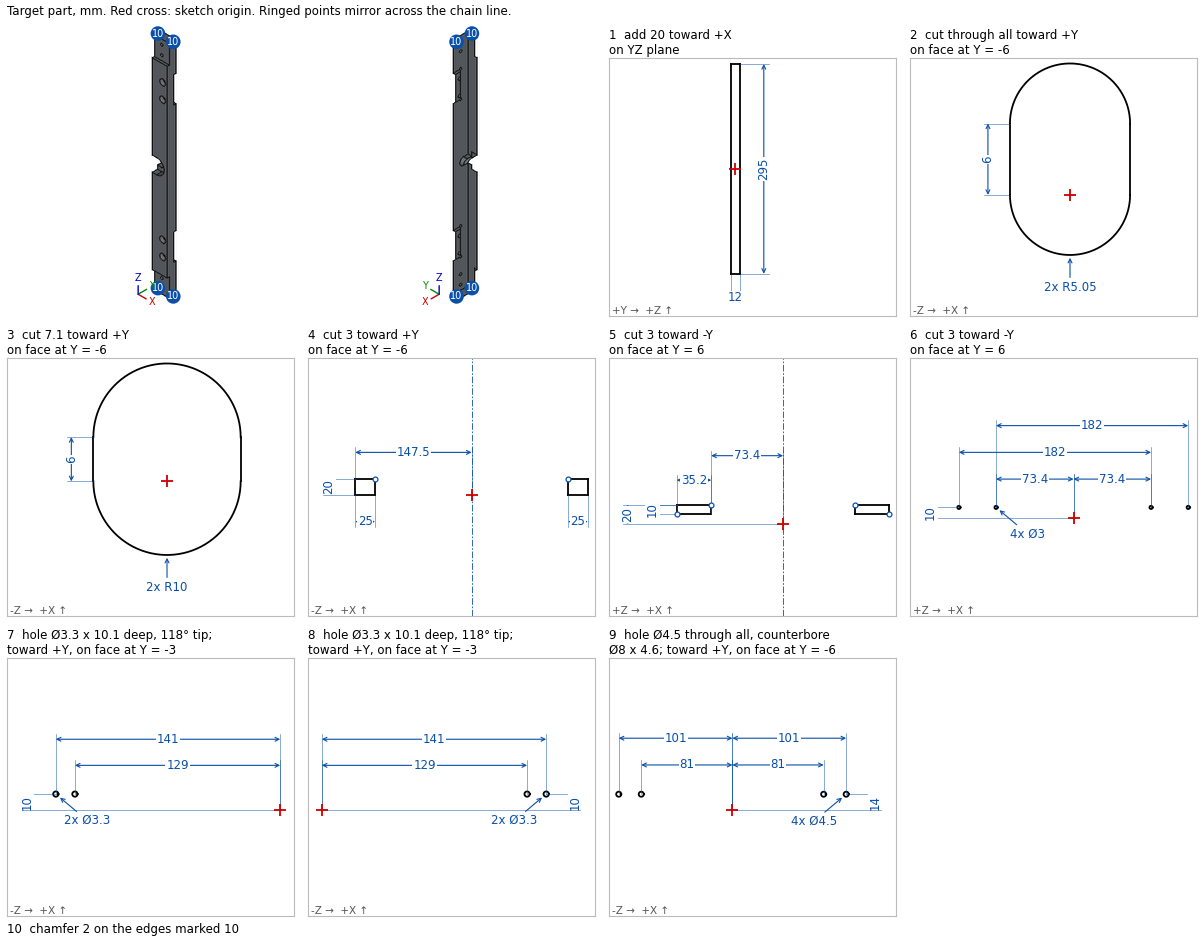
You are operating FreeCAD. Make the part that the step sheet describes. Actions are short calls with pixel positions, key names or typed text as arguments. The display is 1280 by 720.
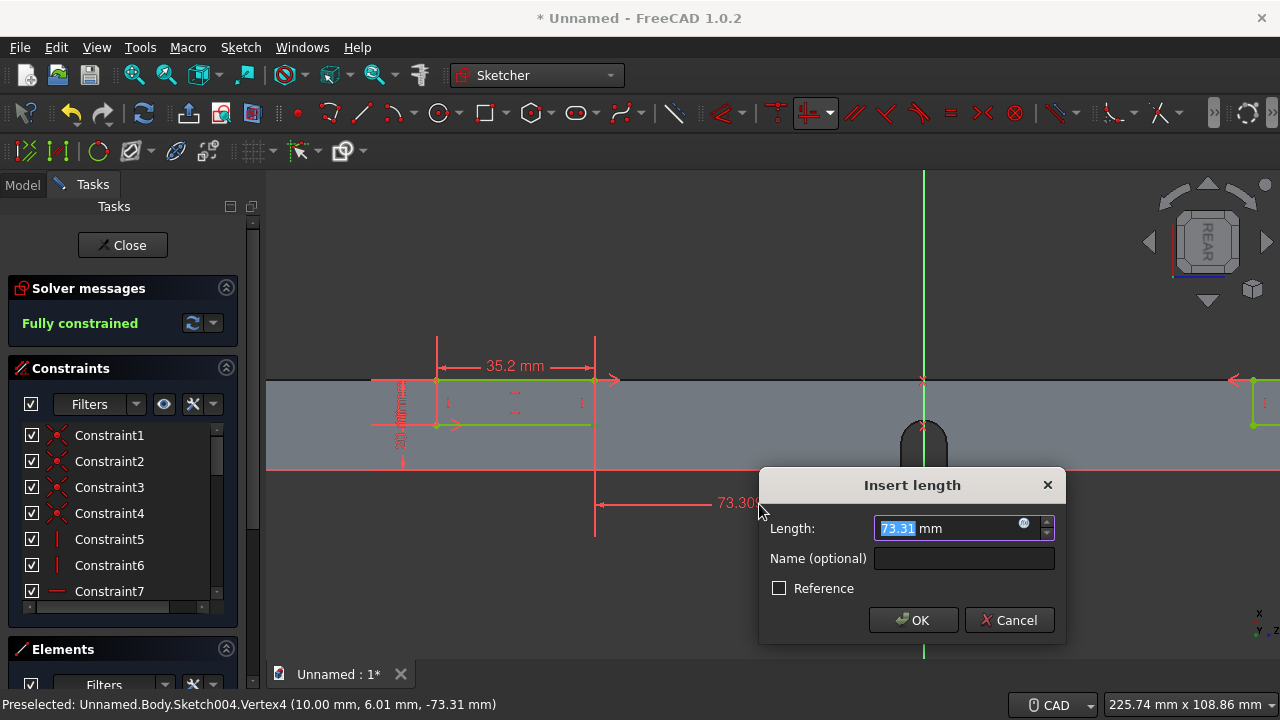
text(73.4)
key(Return)
key(Escape)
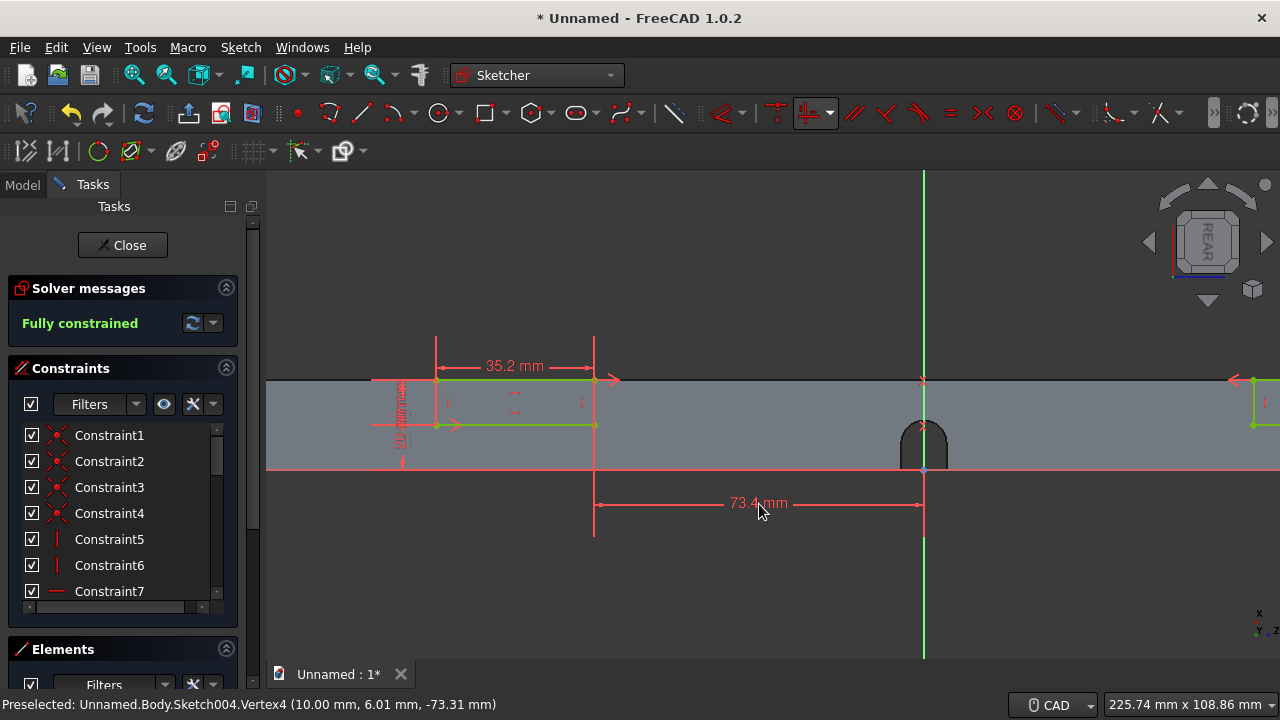
click(123, 245)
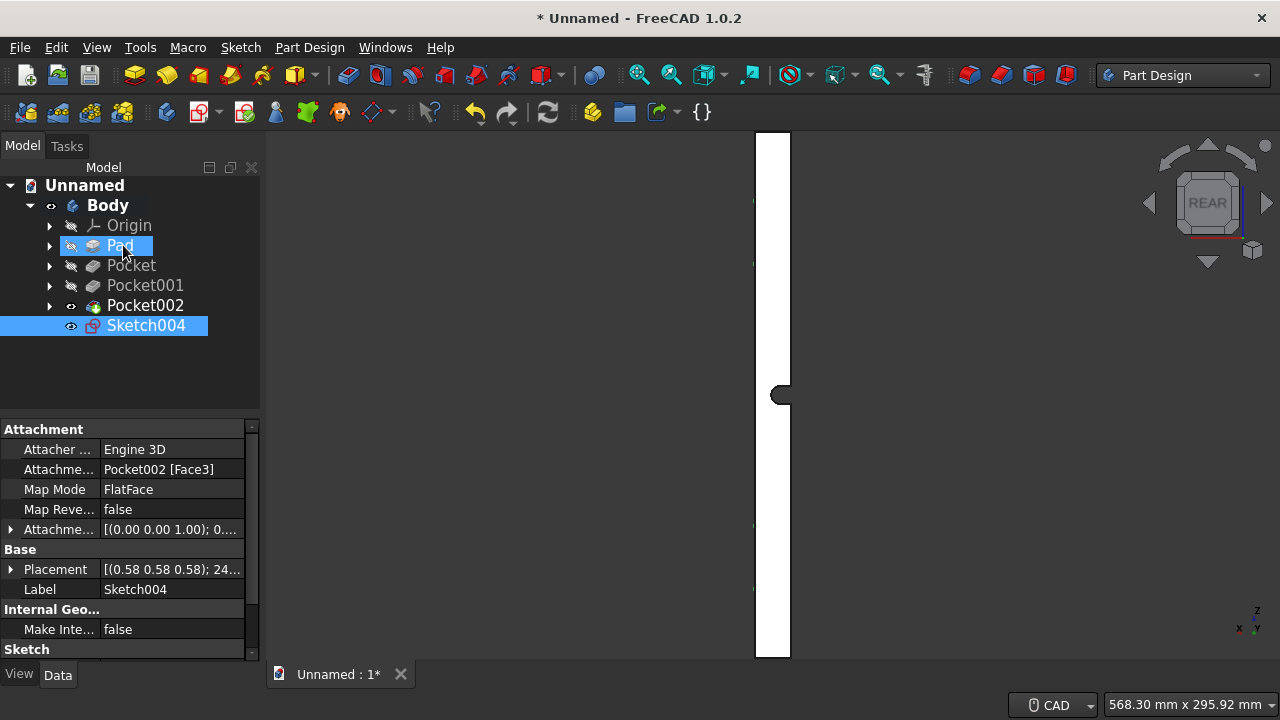
click(350, 76)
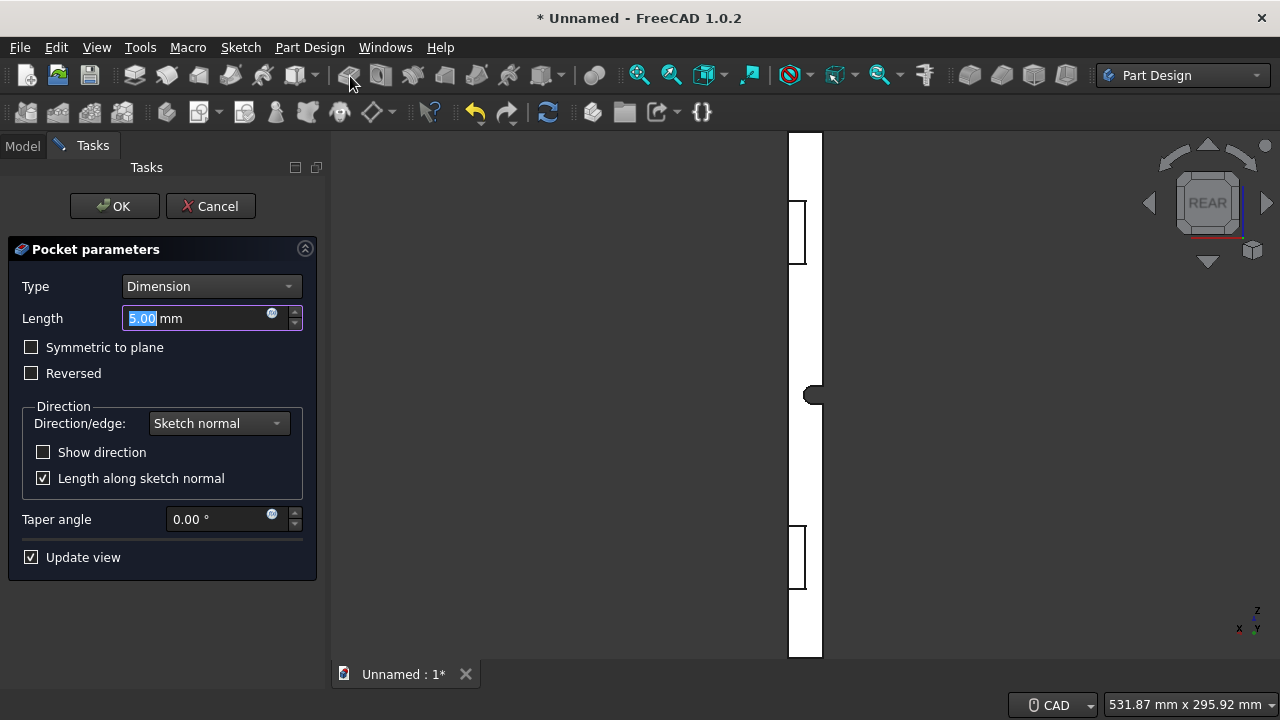
text(3)
key(Tab)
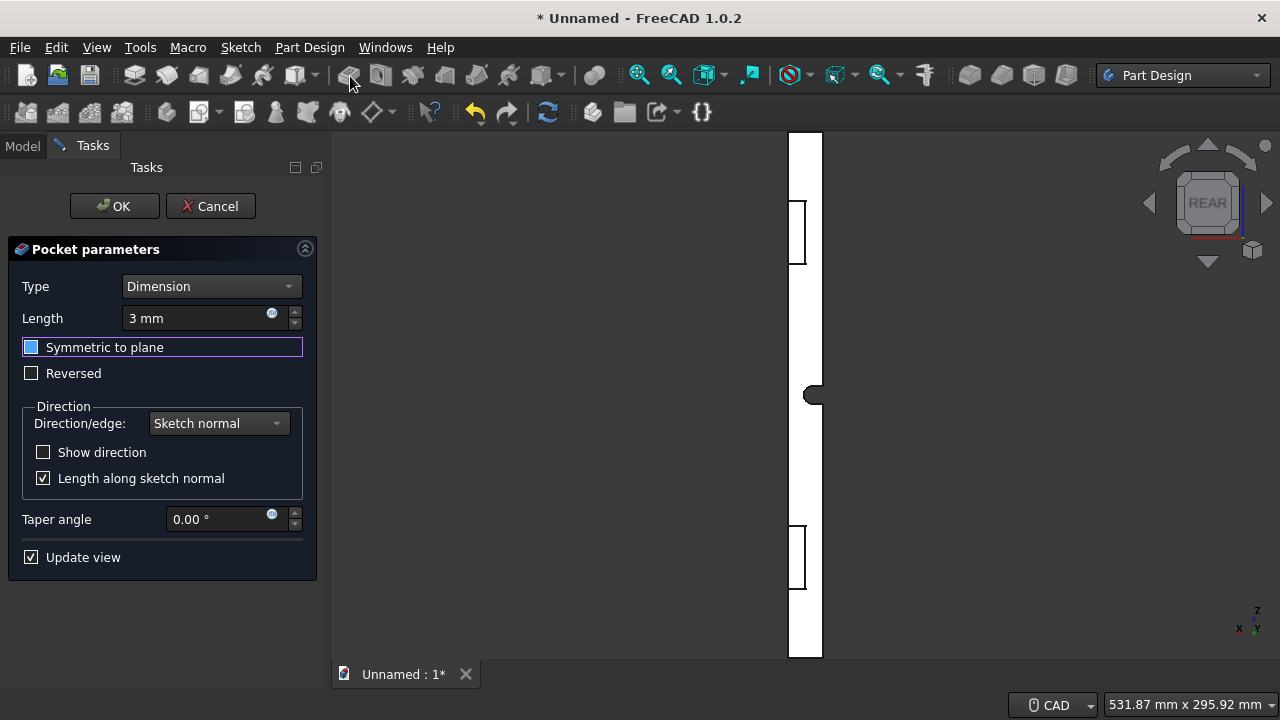
click(115, 206)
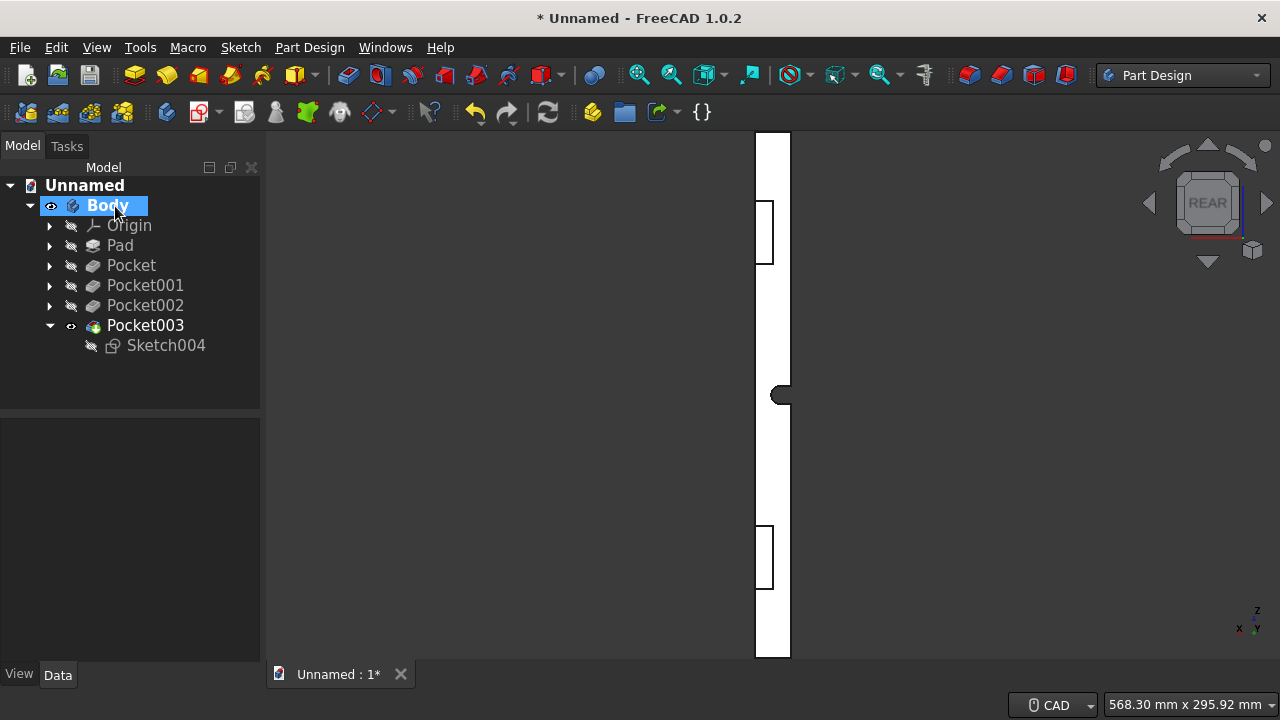
click(773, 469)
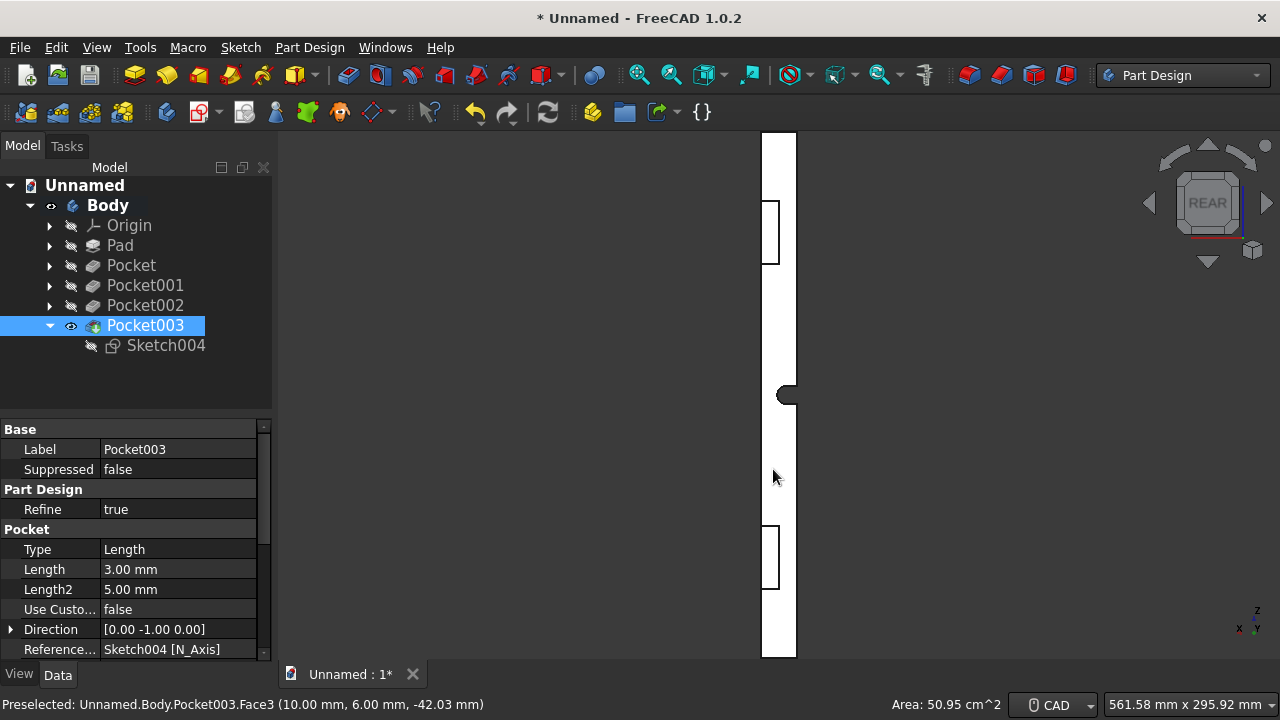
click(200, 112)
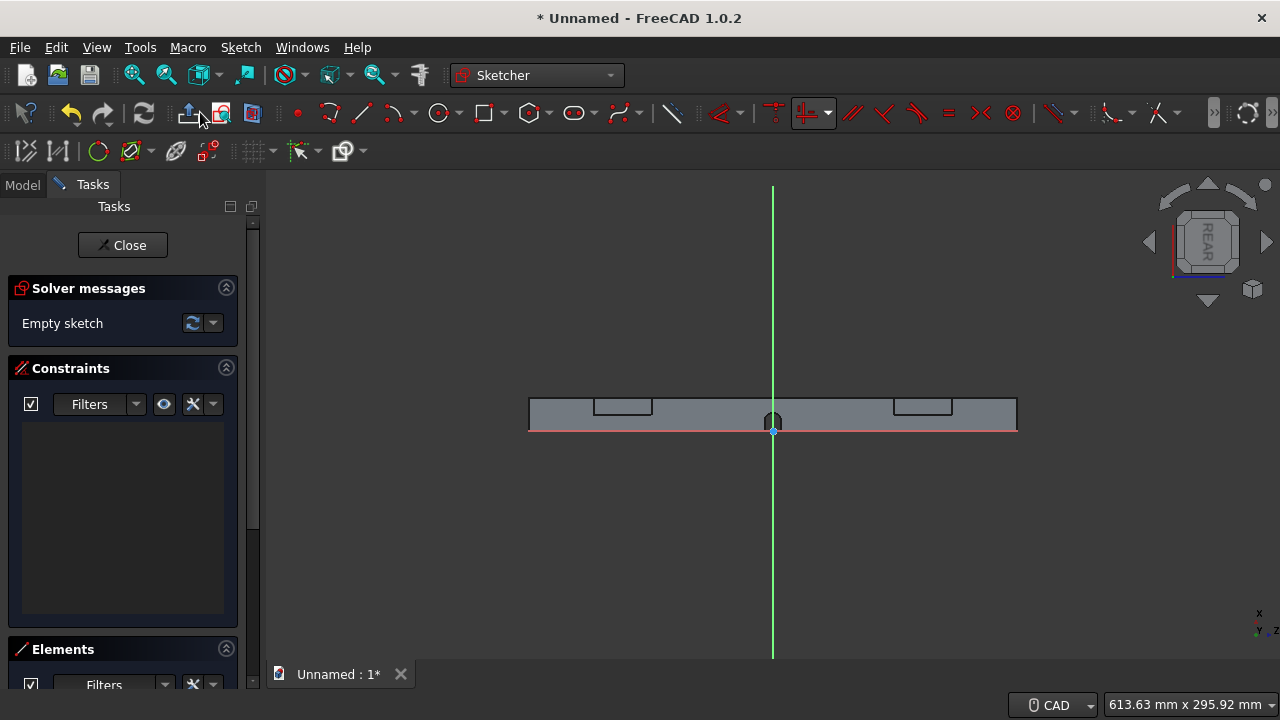
scroll(912, 436, up, 2)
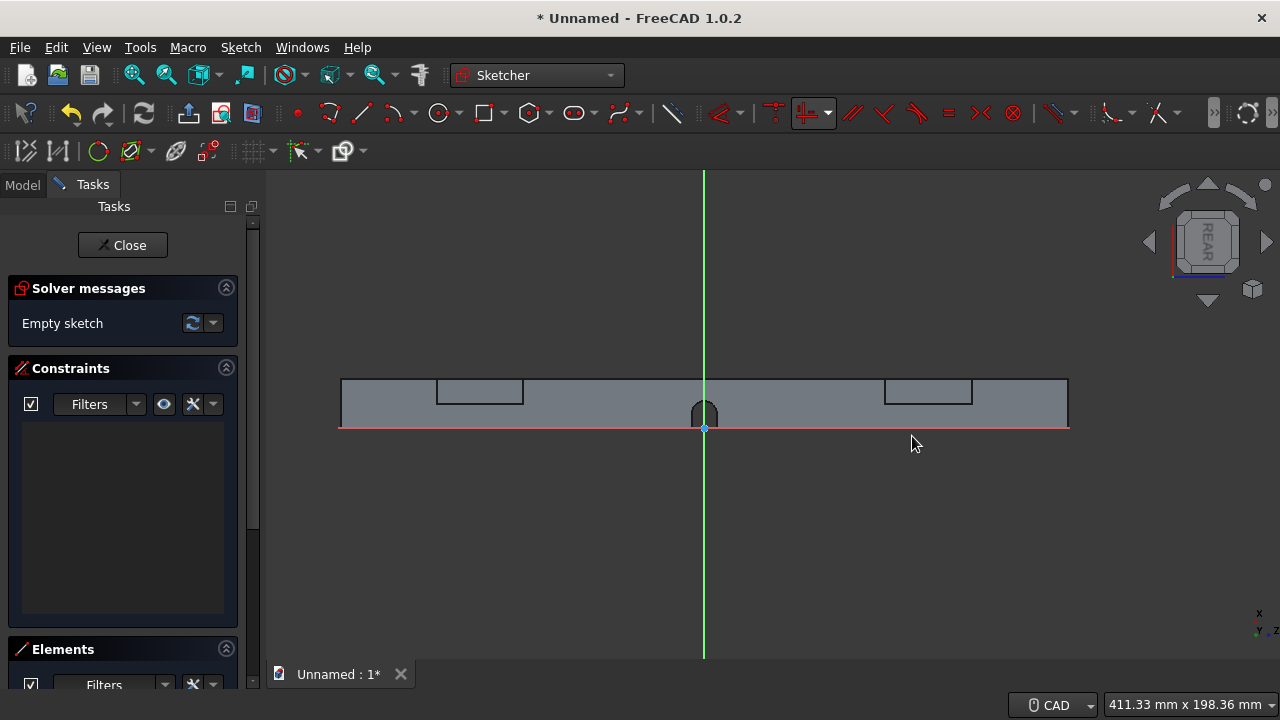
click(440, 114)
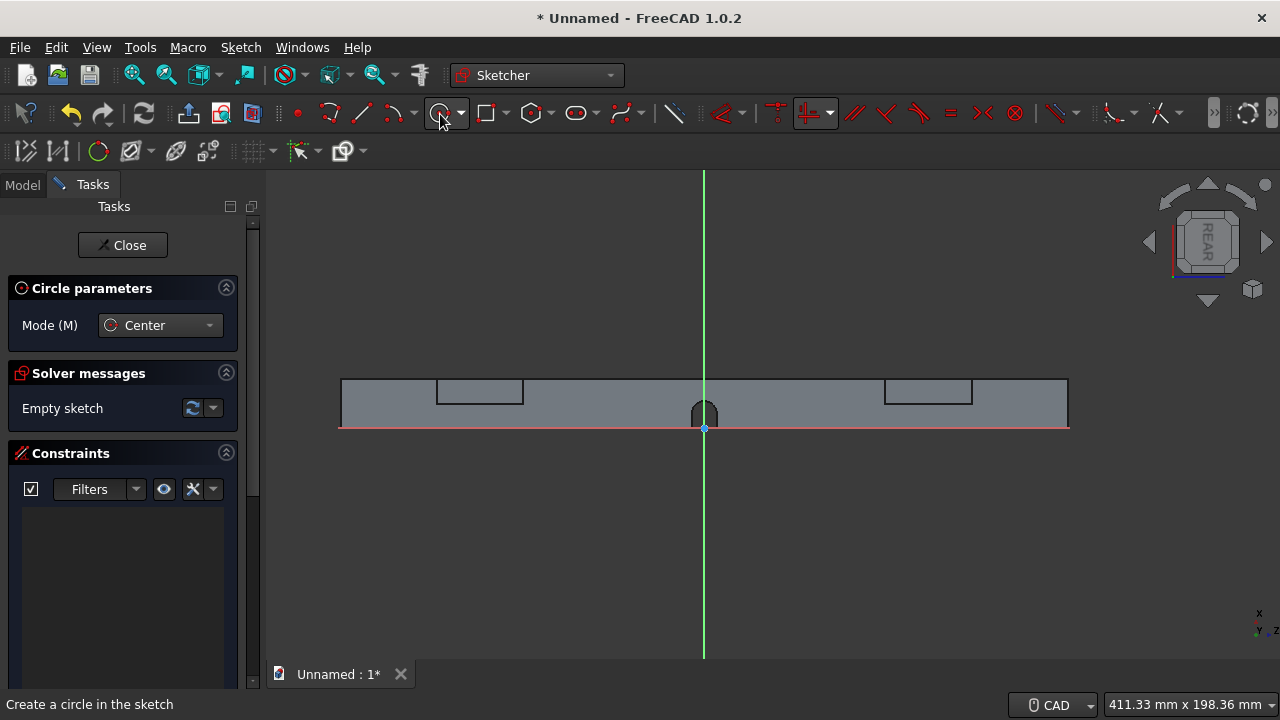
scroll(437, 404, up, 10)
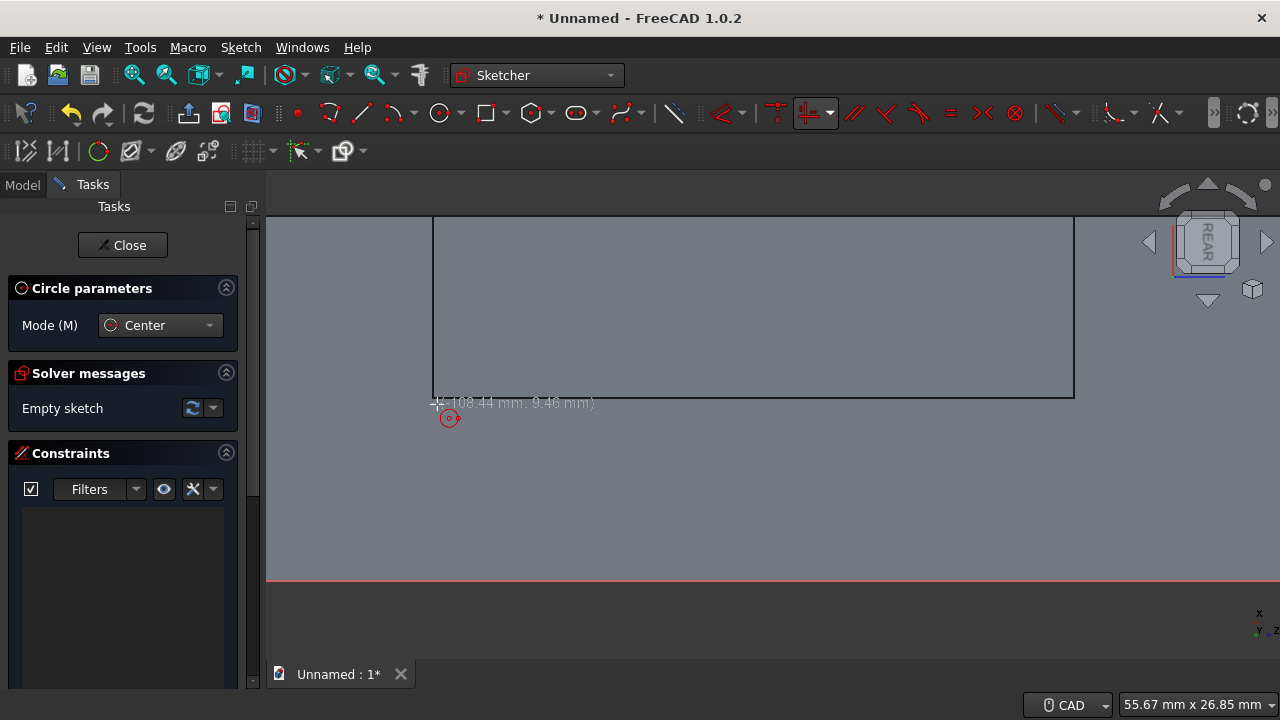
scroll(437, 405, down, 10)